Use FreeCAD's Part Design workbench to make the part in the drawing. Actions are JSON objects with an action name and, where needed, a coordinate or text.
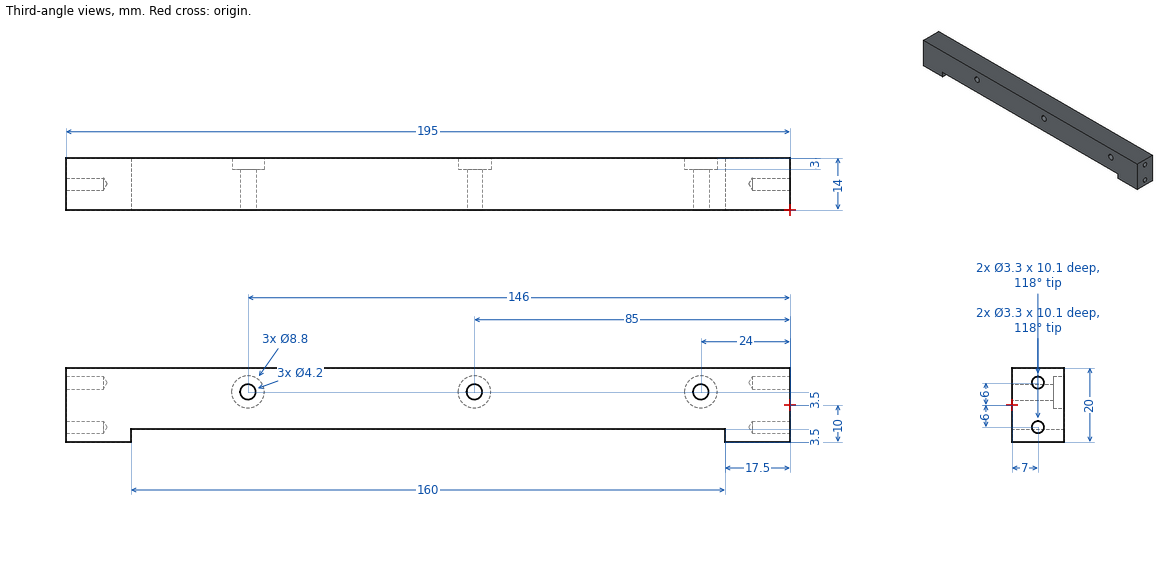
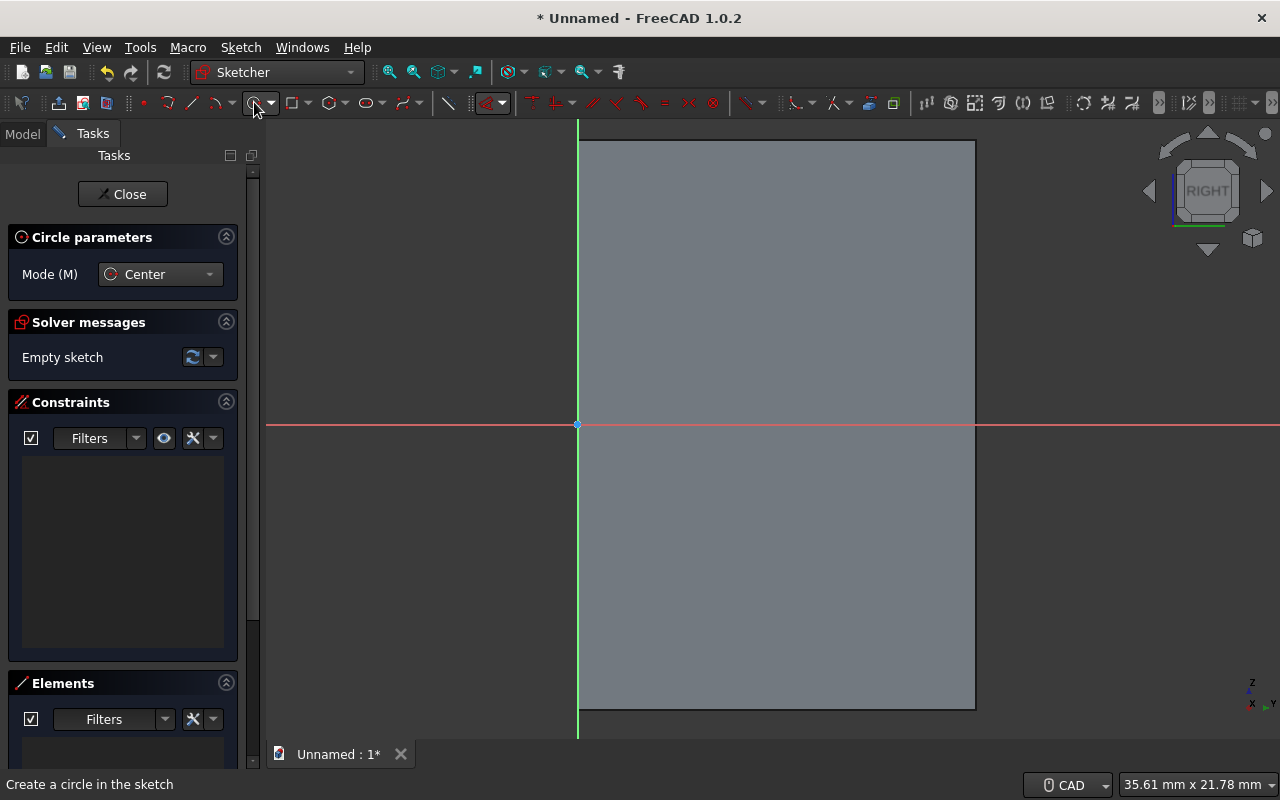
{"action": "left_click", "coordinate": [777, 254]}
{"action": "left_click", "coordinate": [810, 221]}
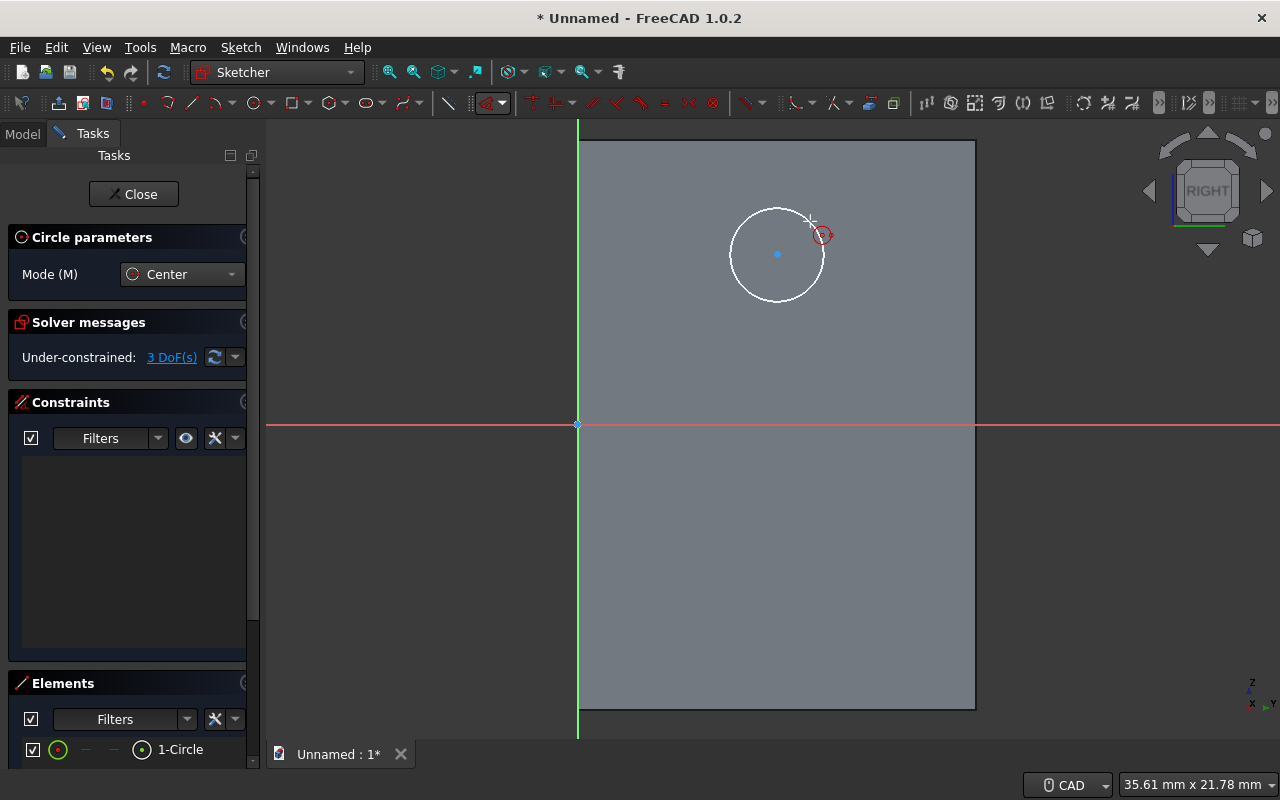
{"action": "left_click", "coordinate": [777, 596]}
{"action": "left_click", "coordinate": [810, 563]}
{"action": "key", "text": "Escape"}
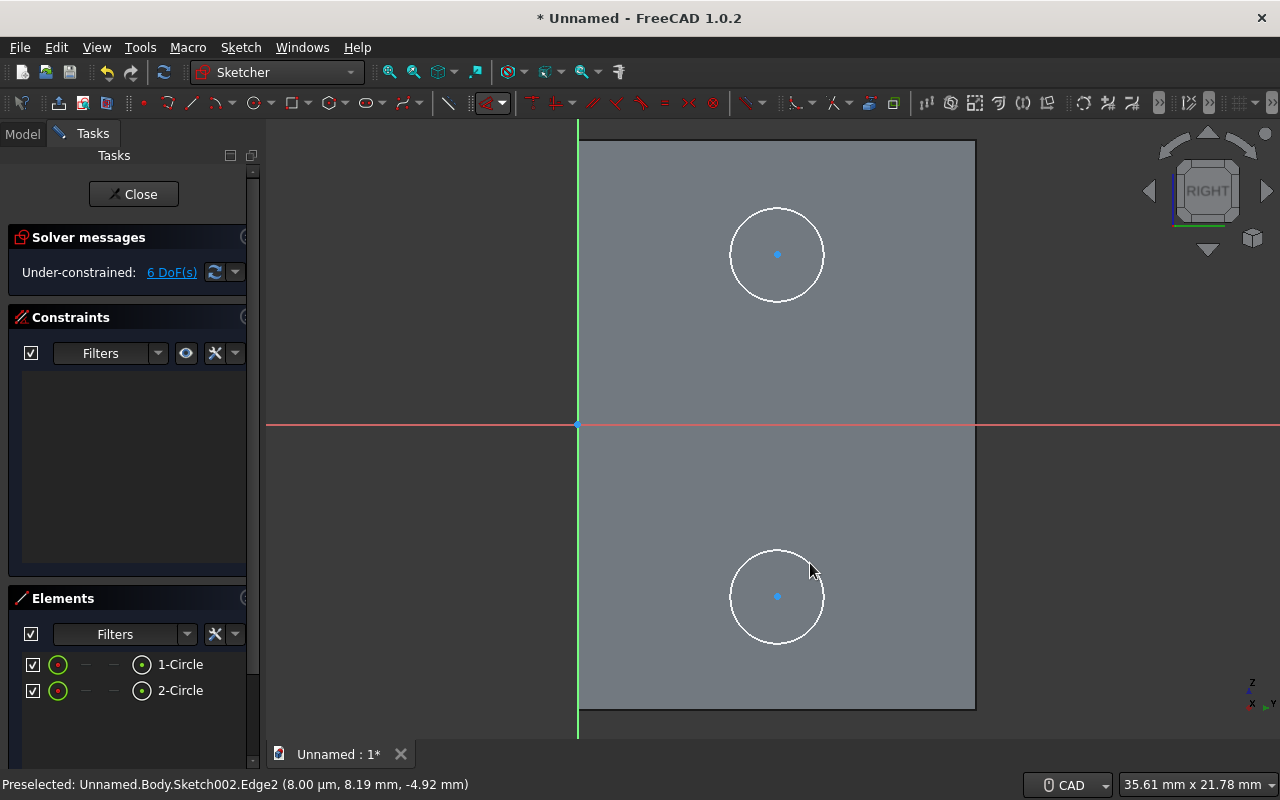
{"action": "left_click", "coordinate": [810, 222]}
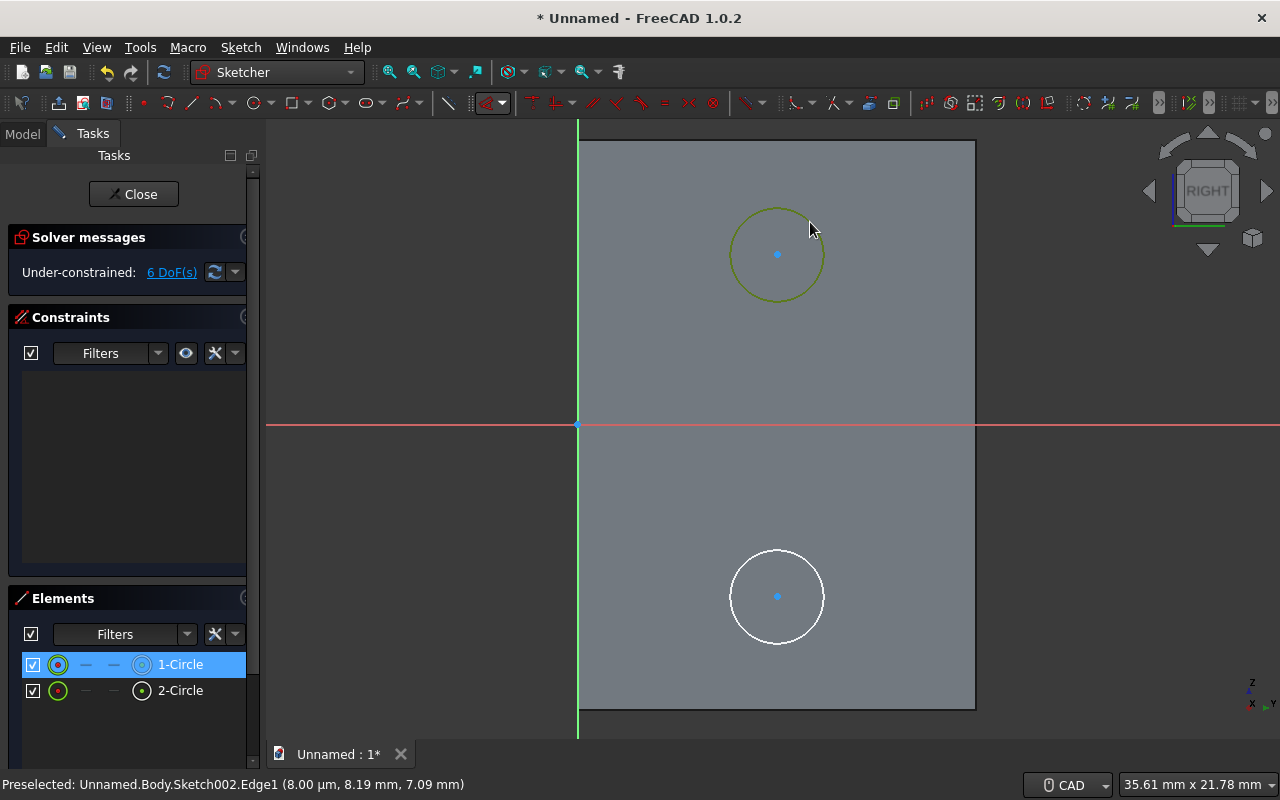
{"action": "left_click", "coordinate": [810, 564]}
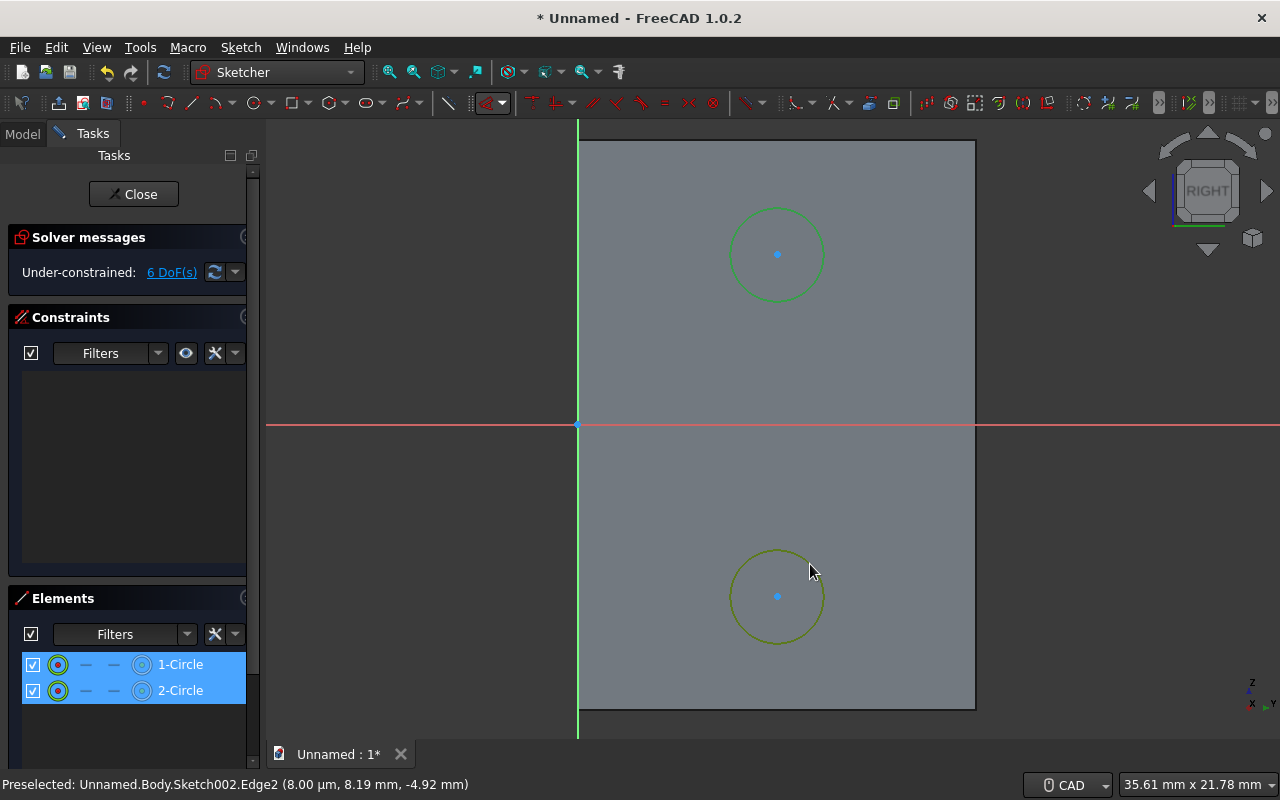
{"action": "key", "text": "e"}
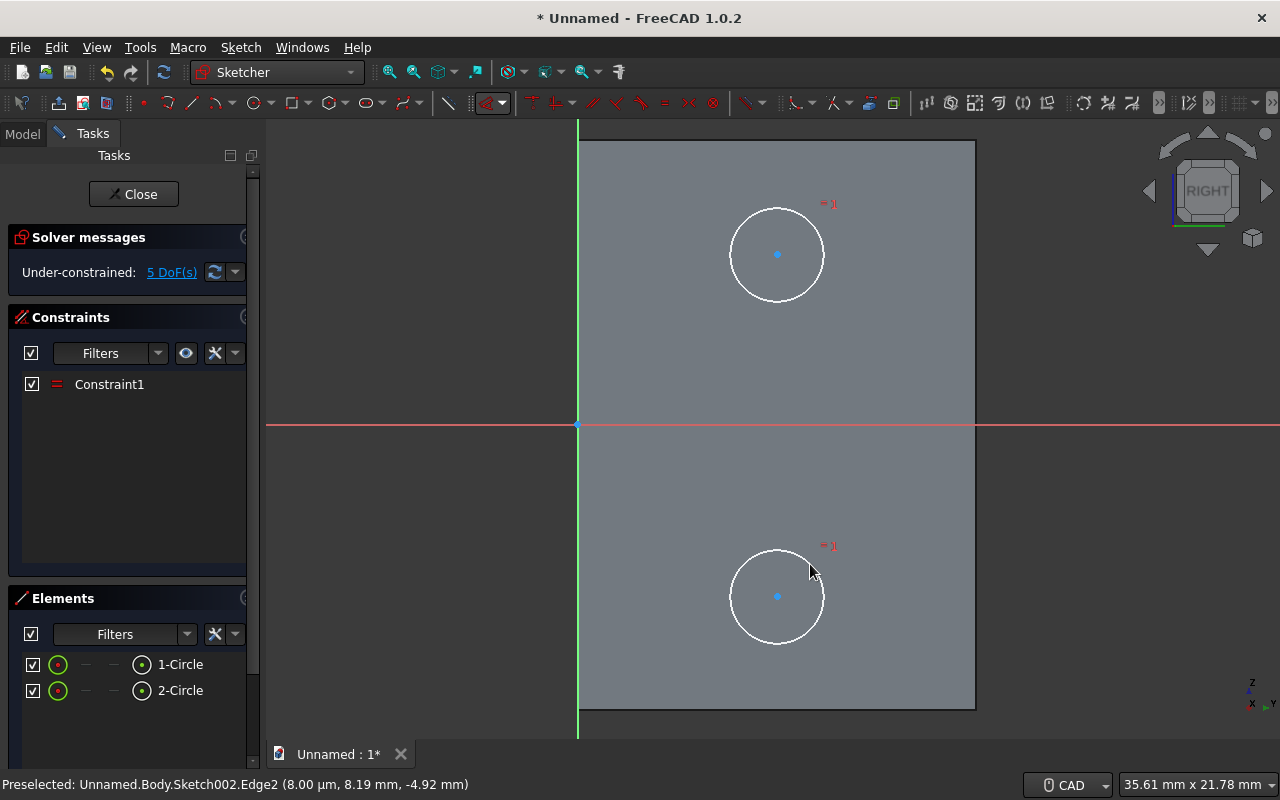
{"action": "left_click", "coordinate": [810, 222]}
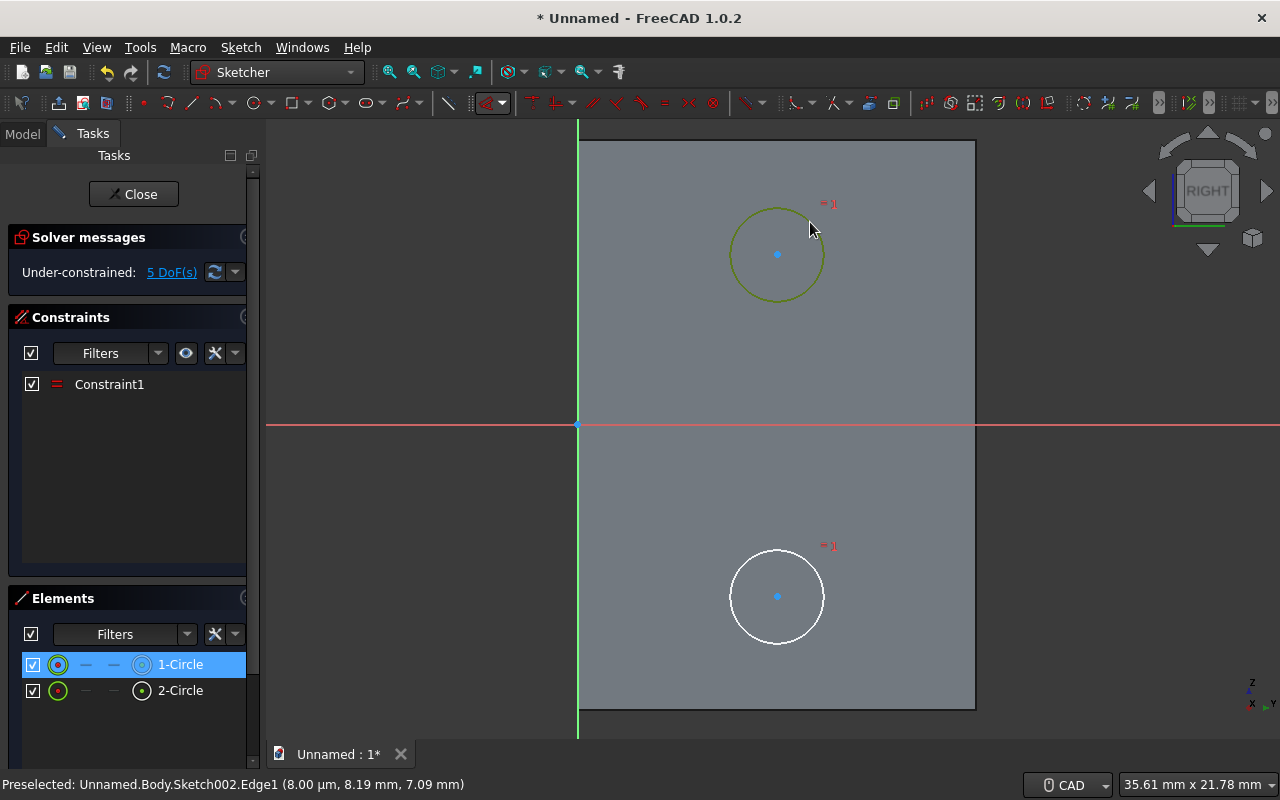
{"action": "key", "text": "k o"}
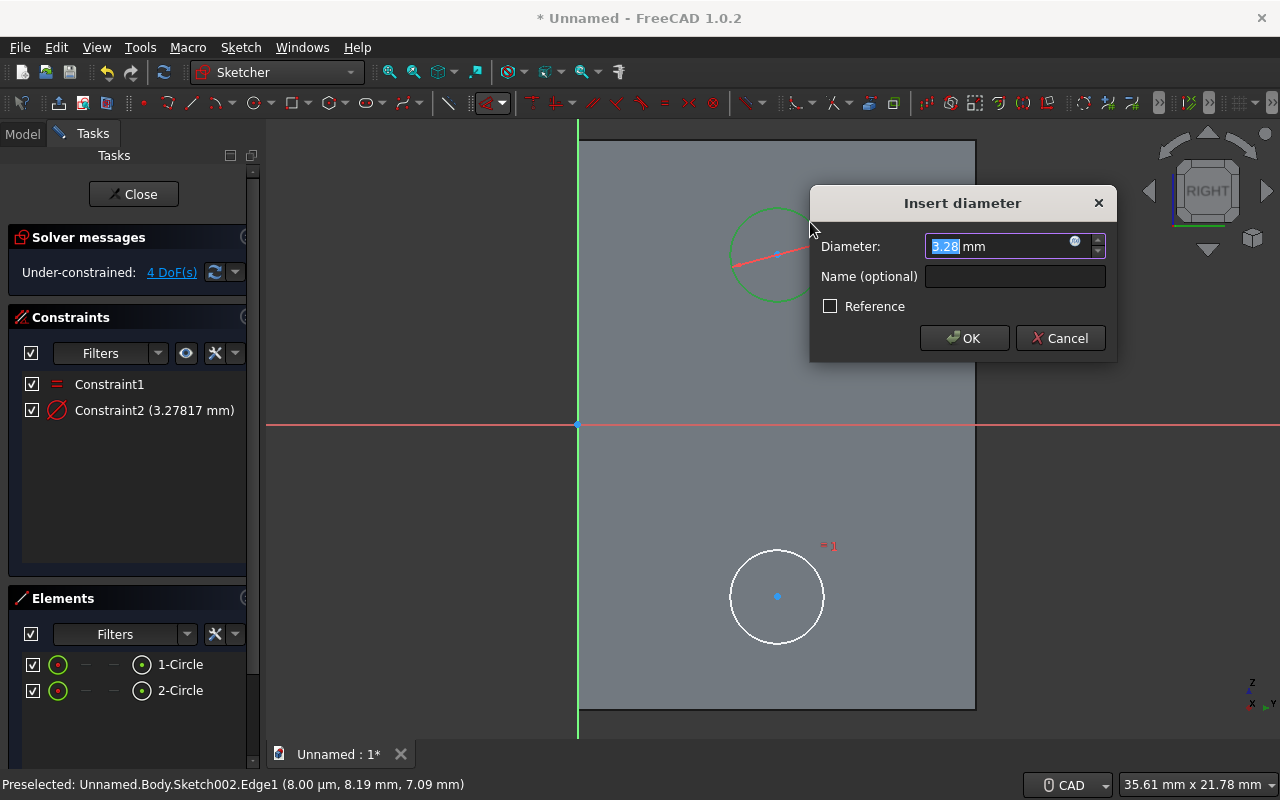
{"action": "type", "text": "3.3"}
{"action": "key", "text": "Return"}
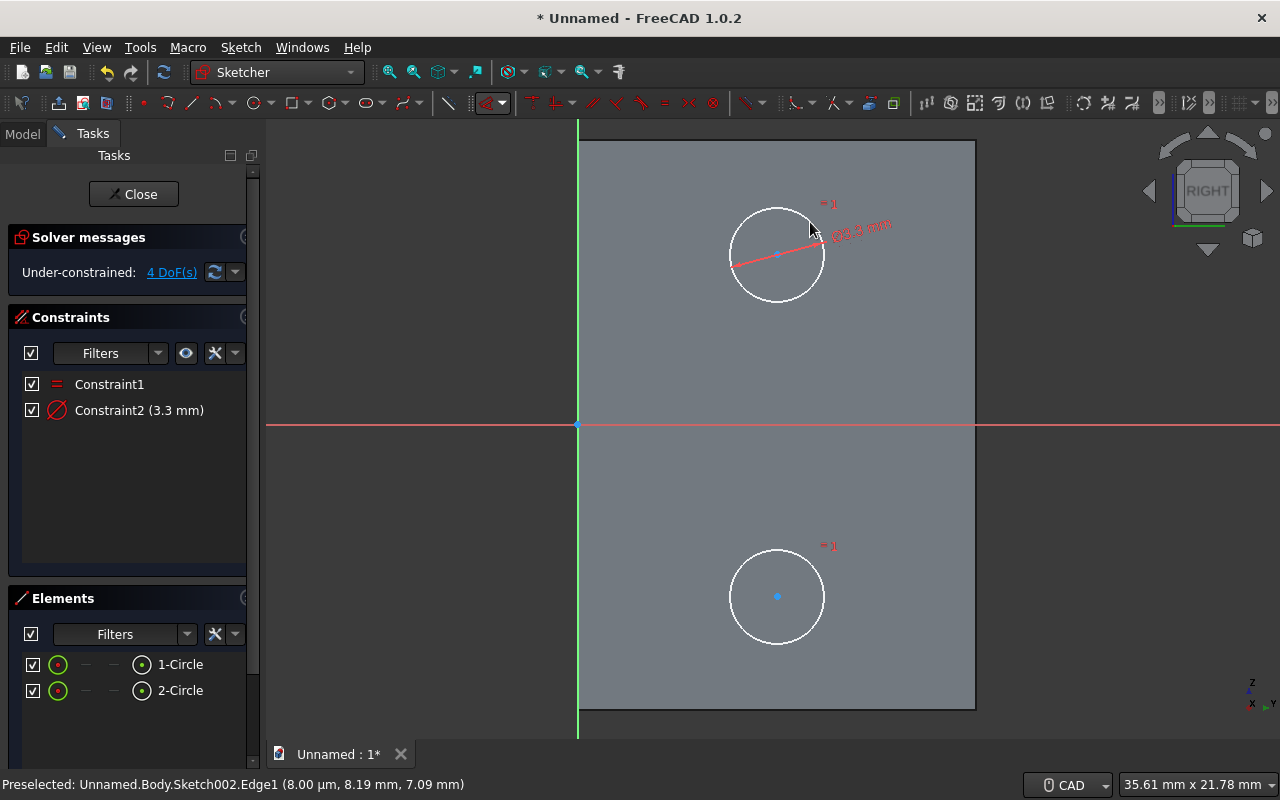
{"action": "left_click", "coordinate": [777, 255]}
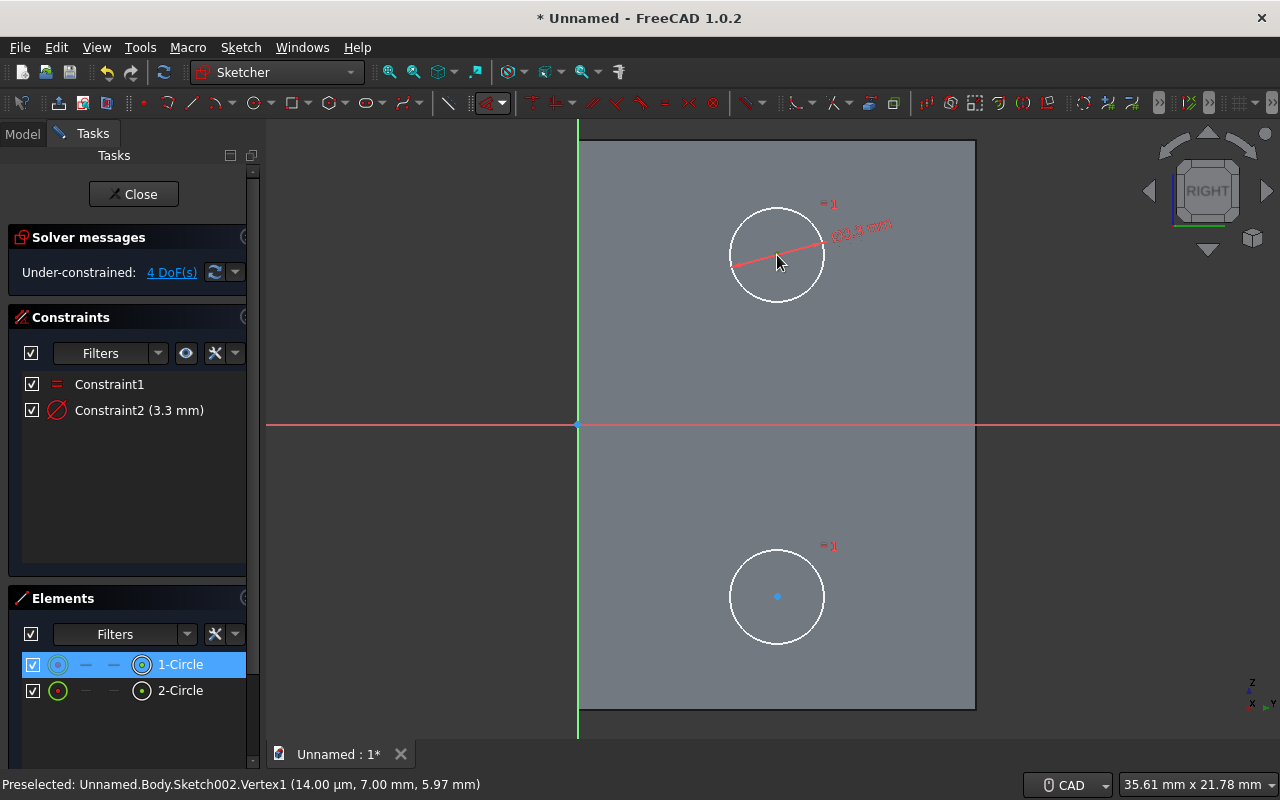
{"action": "key", "text": "l"}